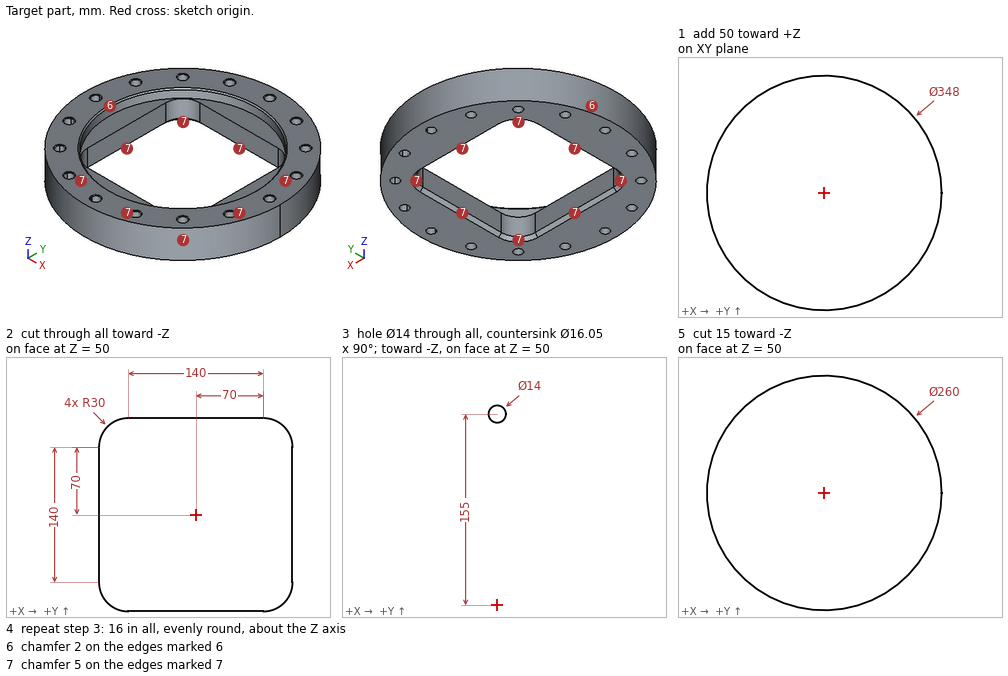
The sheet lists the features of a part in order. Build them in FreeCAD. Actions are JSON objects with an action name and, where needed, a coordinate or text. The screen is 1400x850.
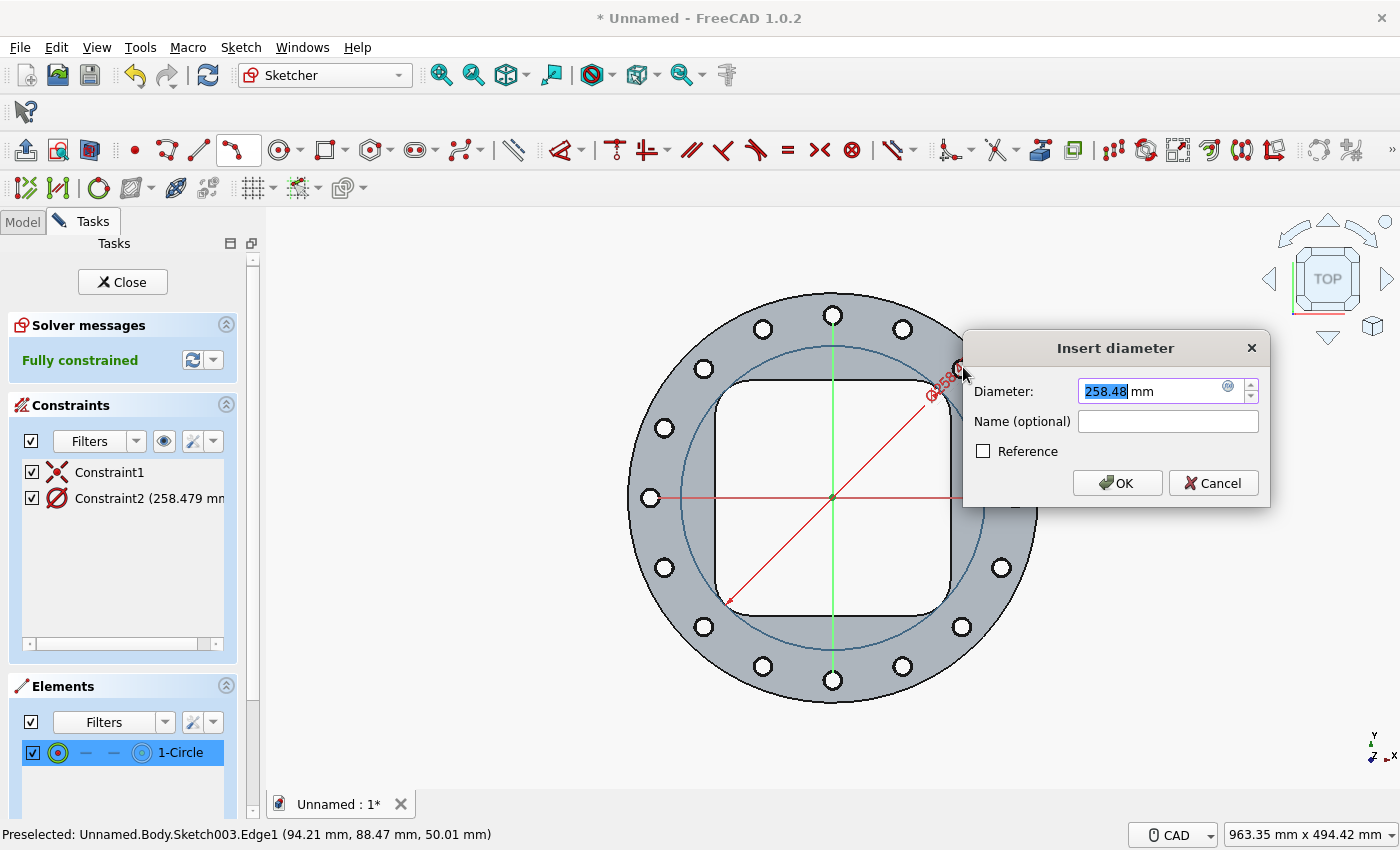
{"action": "type", "text": "260"}
{"action": "key", "text": "Return"}
{"action": "key", "text": "Escape"}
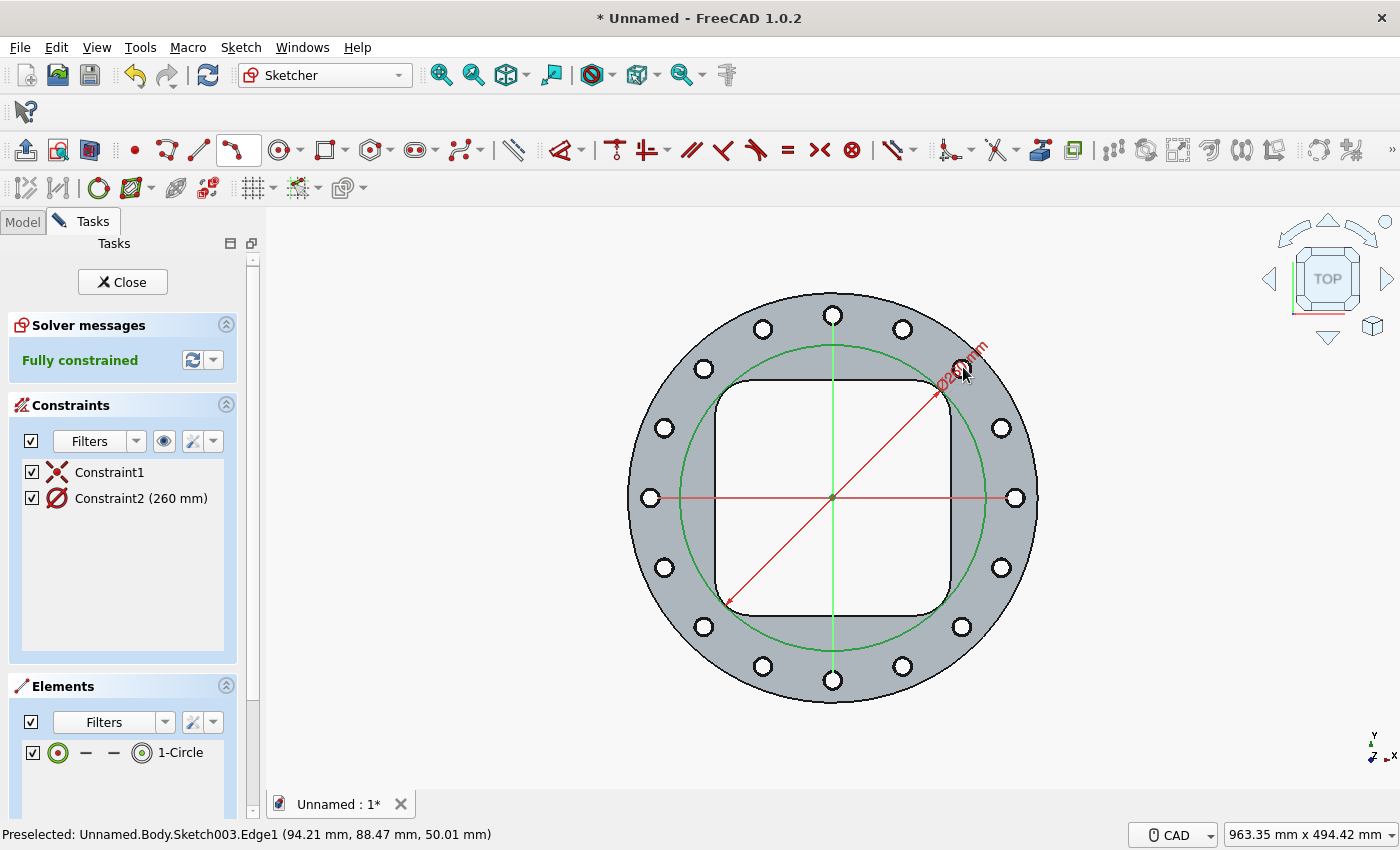
{"action": "left_click", "coordinate": [123, 282]}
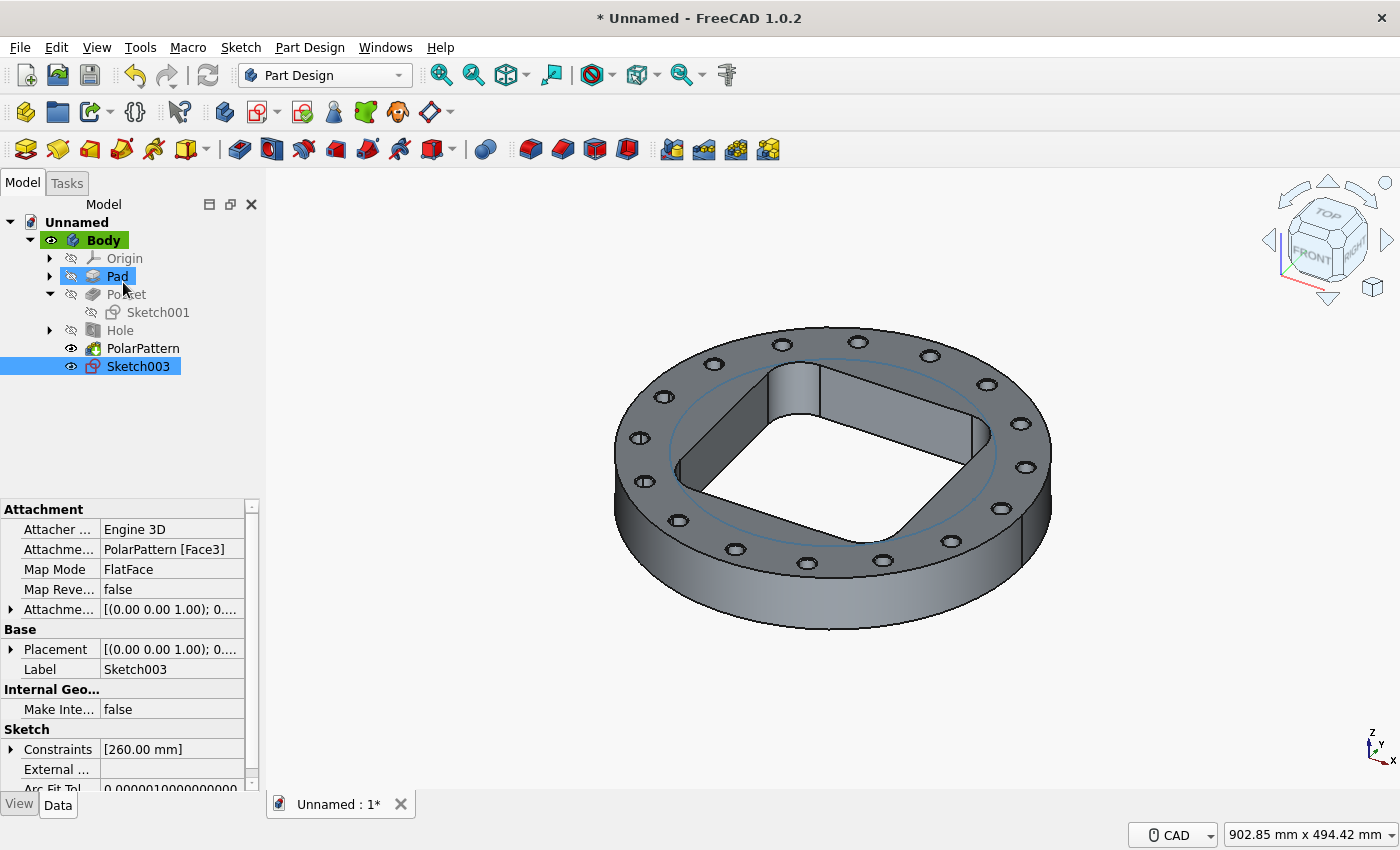
{"action": "left_click", "coordinate": [240, 150]}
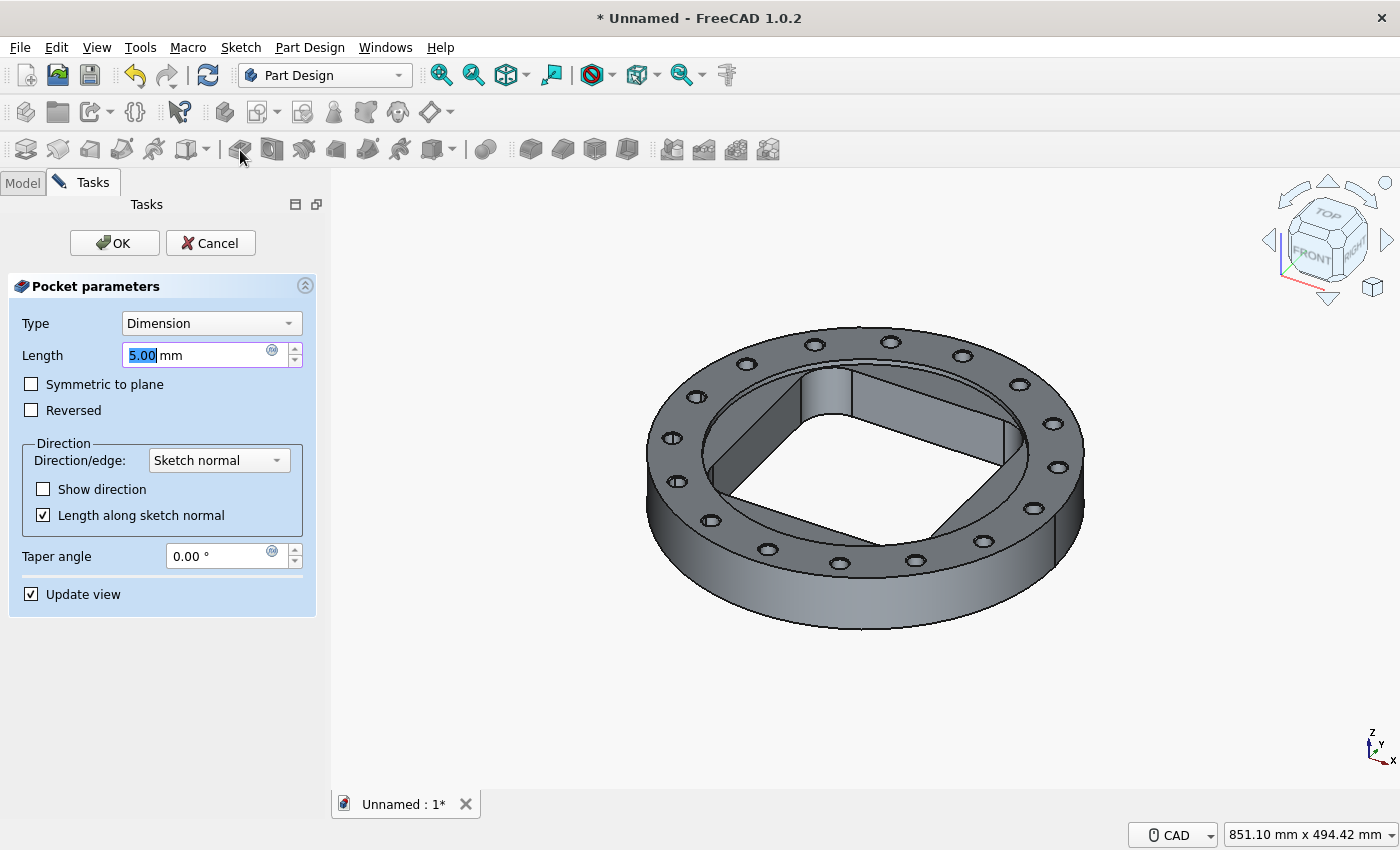
{"action": "type", "text": "15"}
{"action": "key", "text": "Tab"}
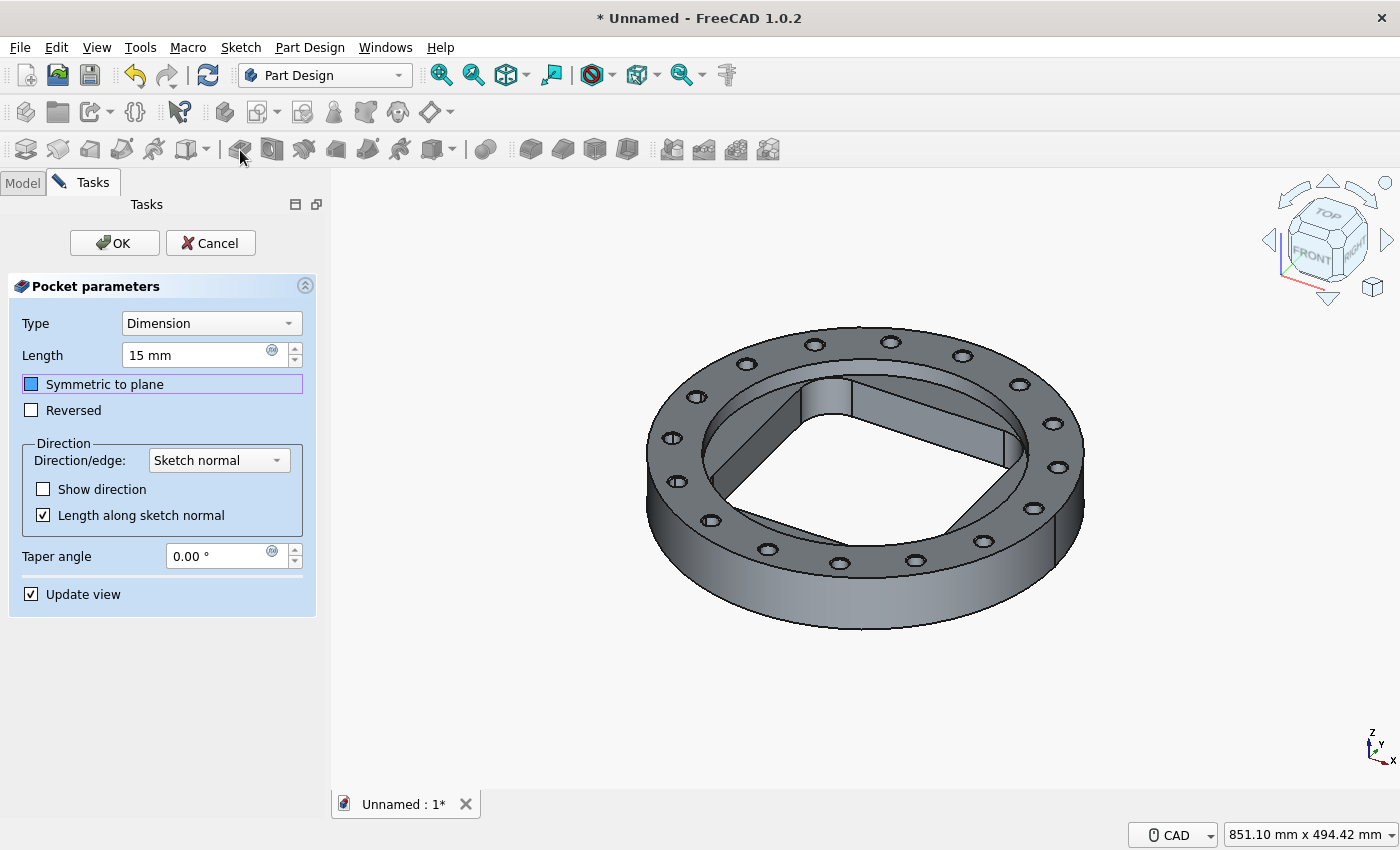
{"action": "left_click", "coordinate": [115, 243]}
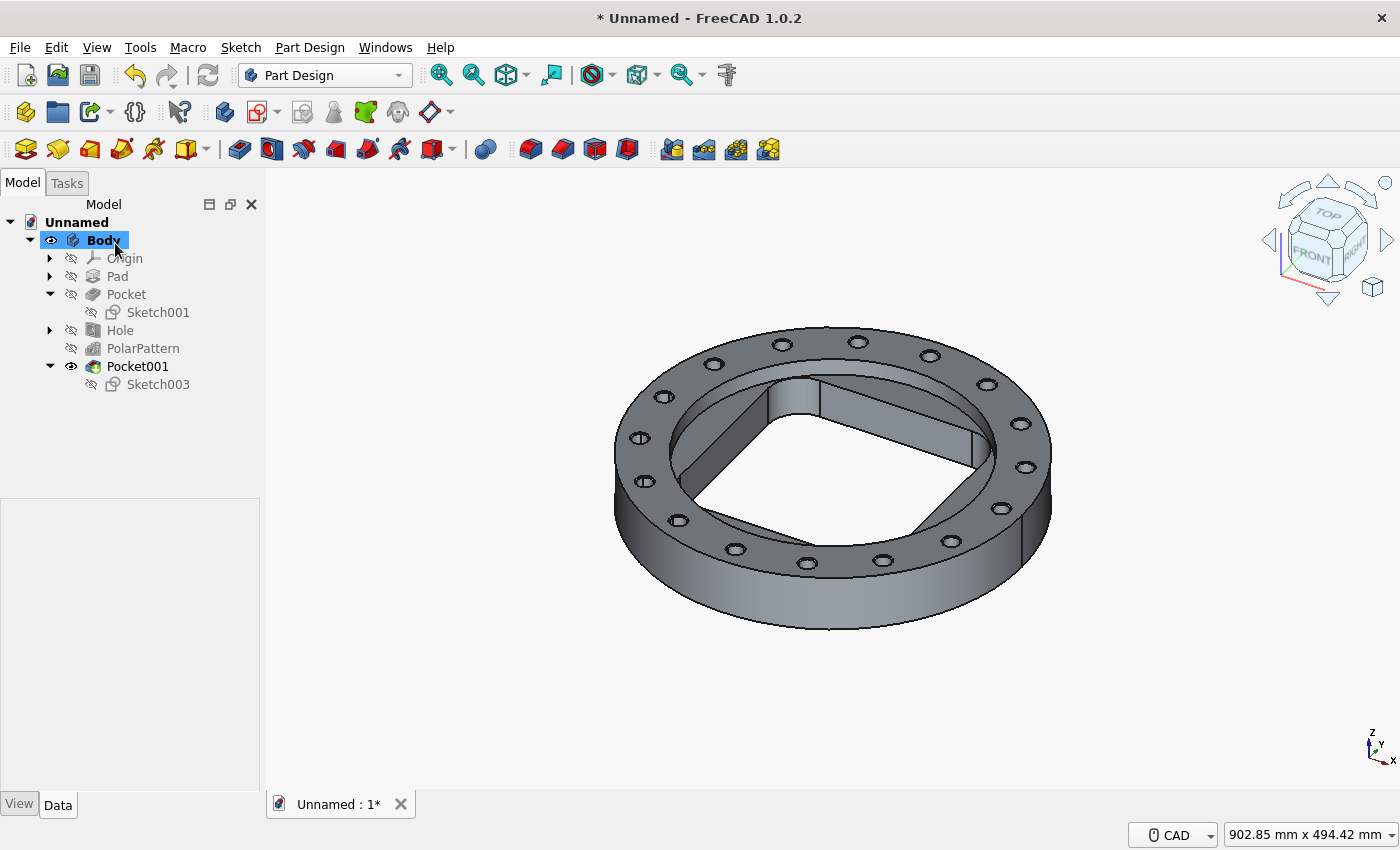
{"action": "left_click", "coordinate": [691, 405]}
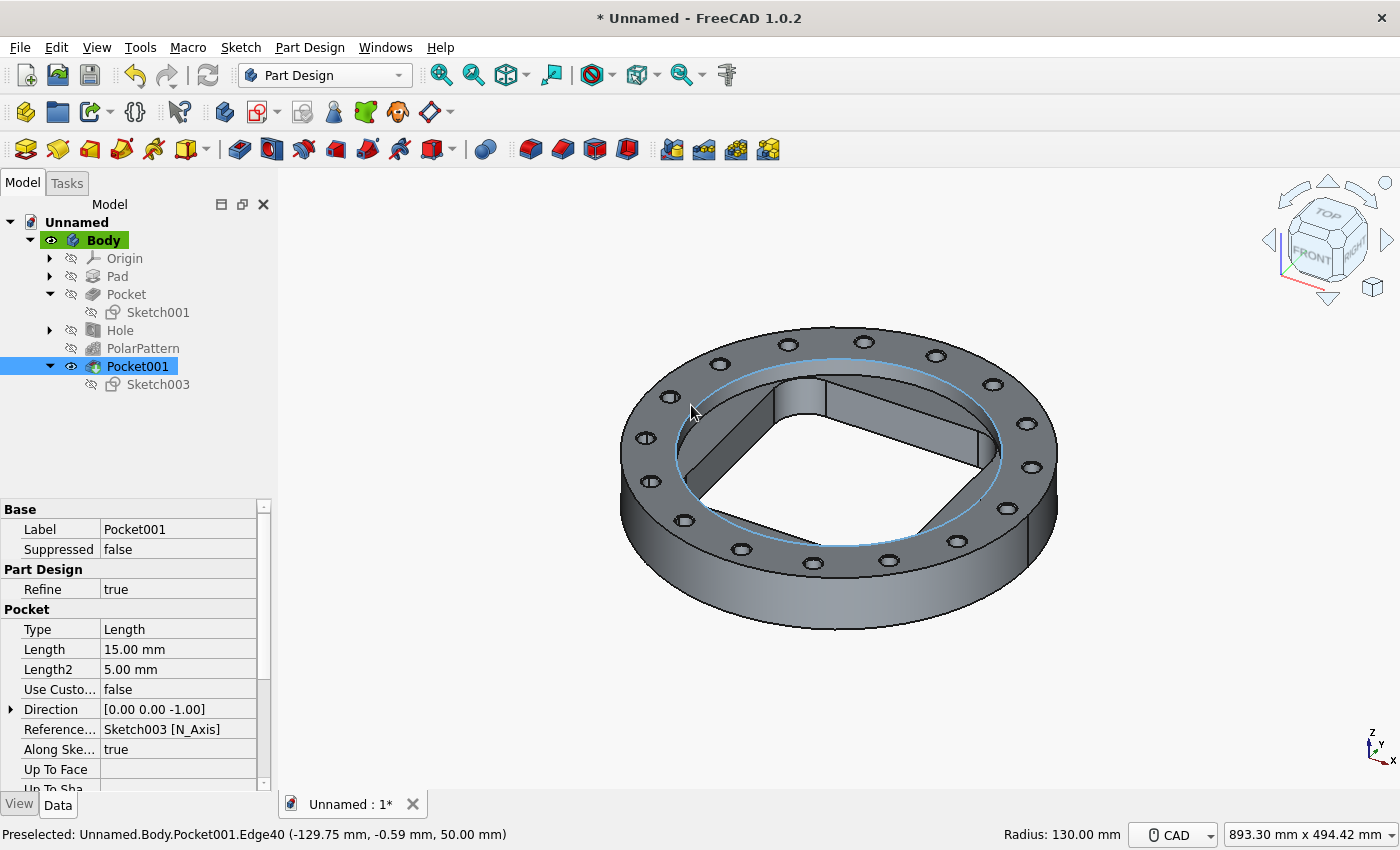
{"action": "left_click", "coordinate": [564, 150]}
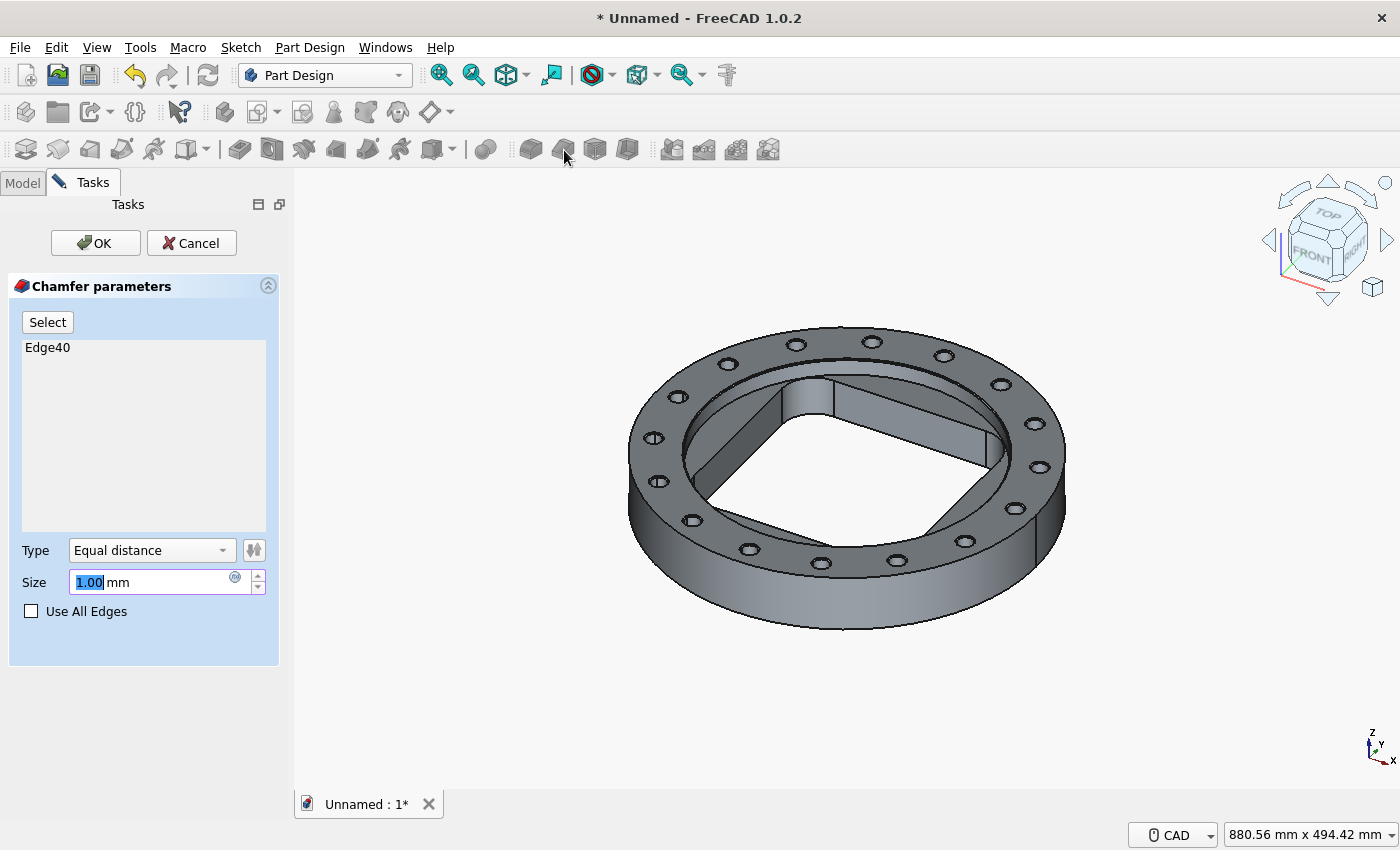
{"action": "type", "text": "2"}
{"action": "key", "text": "Tab"}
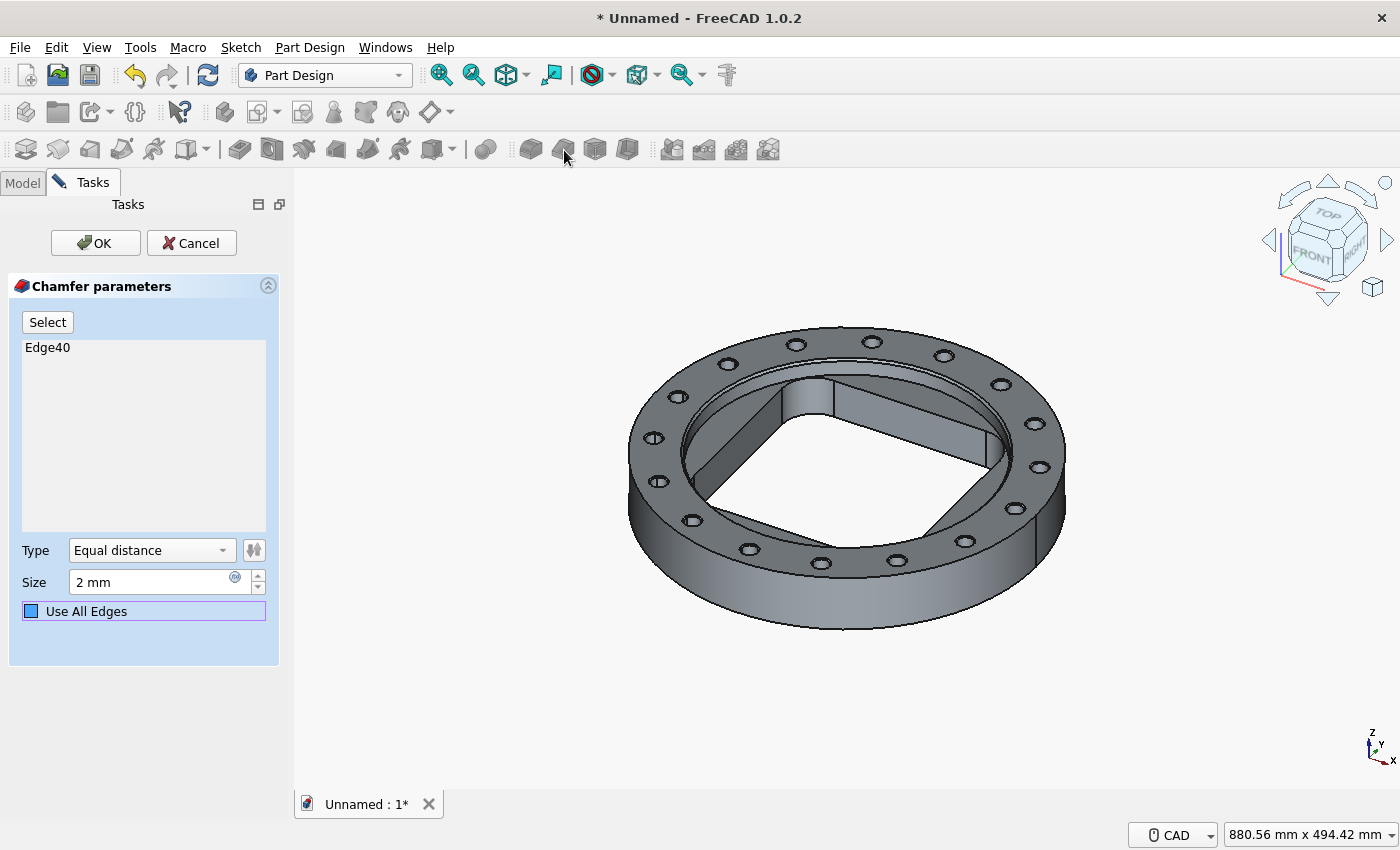
{"action": "left_click", "coordinate": [96, 243]}